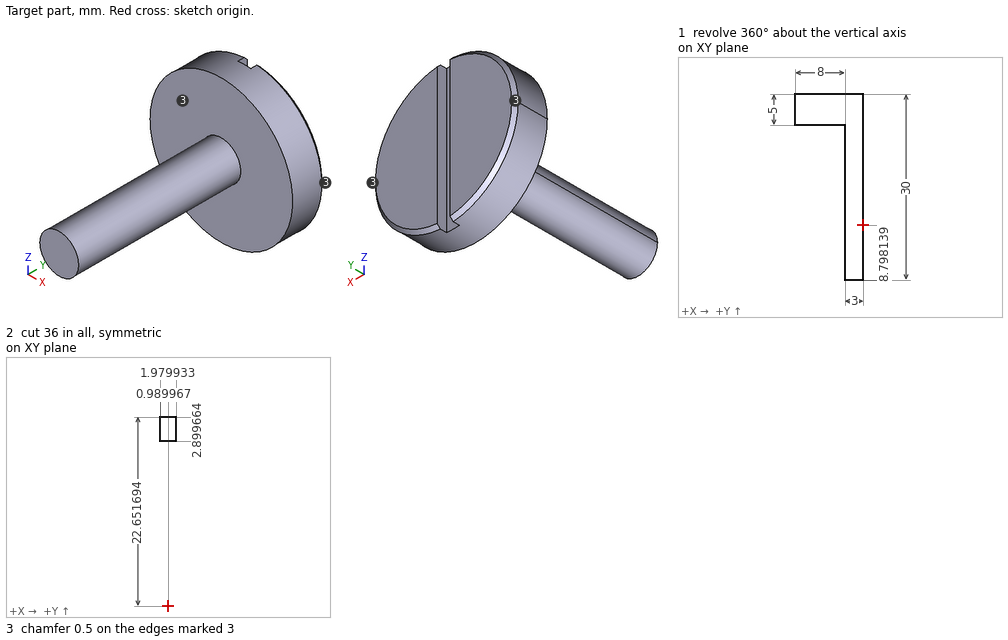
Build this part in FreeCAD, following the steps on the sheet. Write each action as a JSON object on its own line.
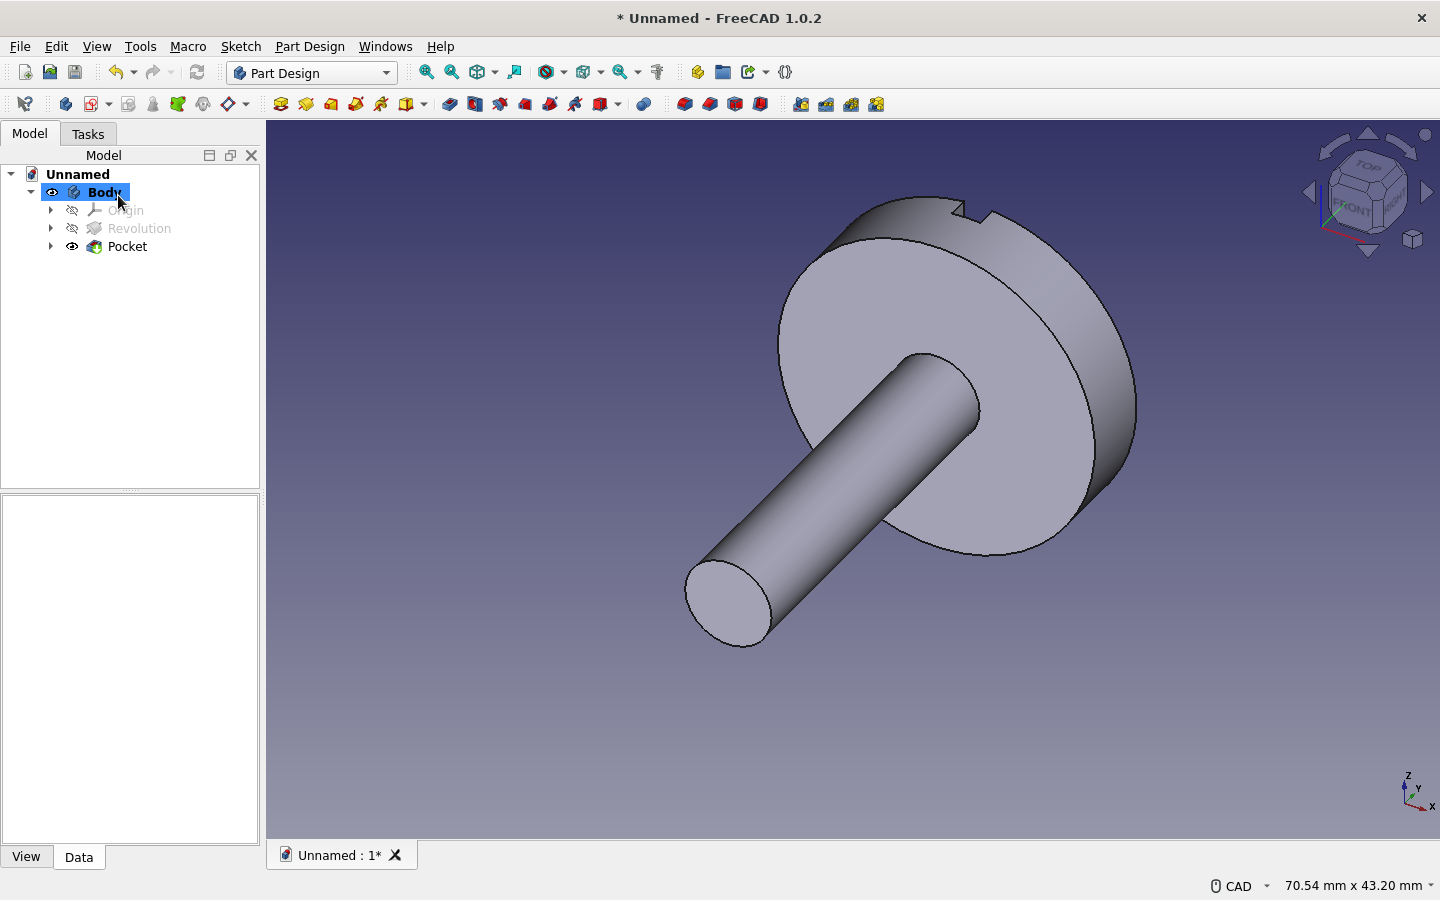
{"action": "key", "text": "0"}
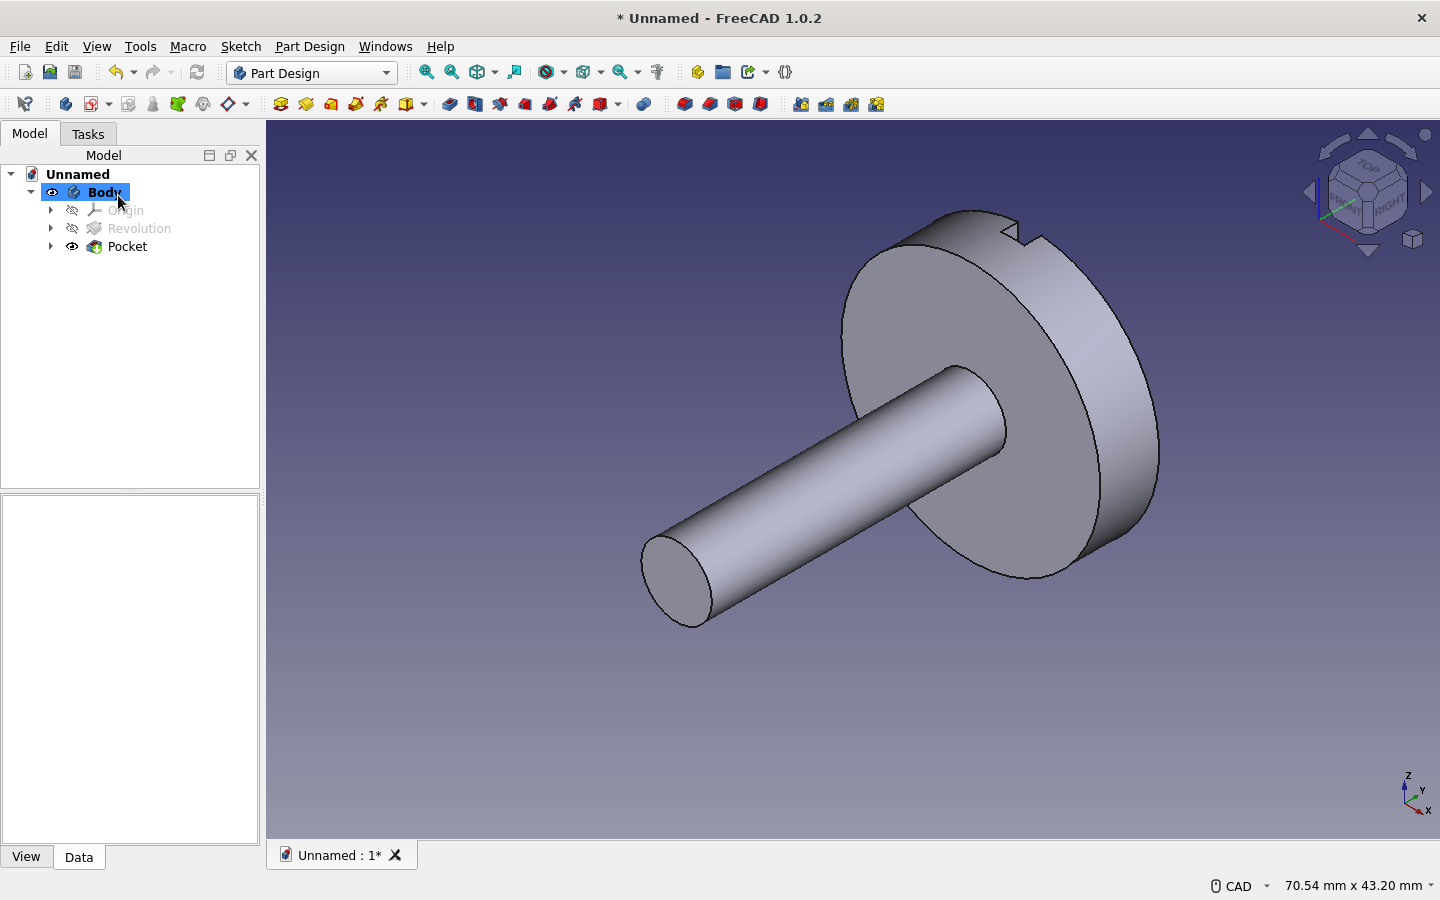
{"action": "key", "text": "2"}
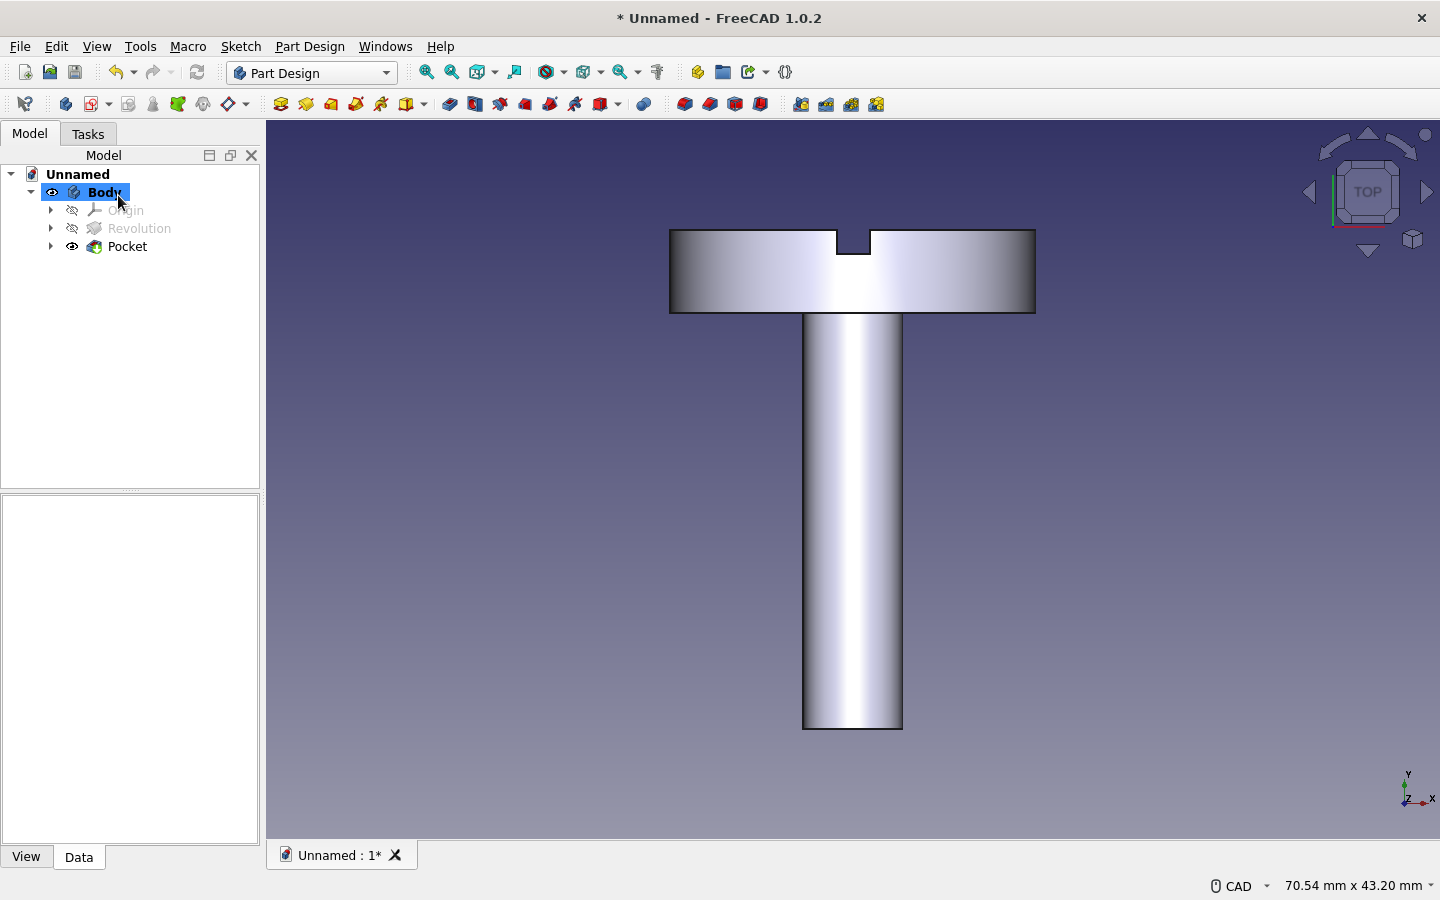
{"action": "left_click", "coordinate": [886, 229]}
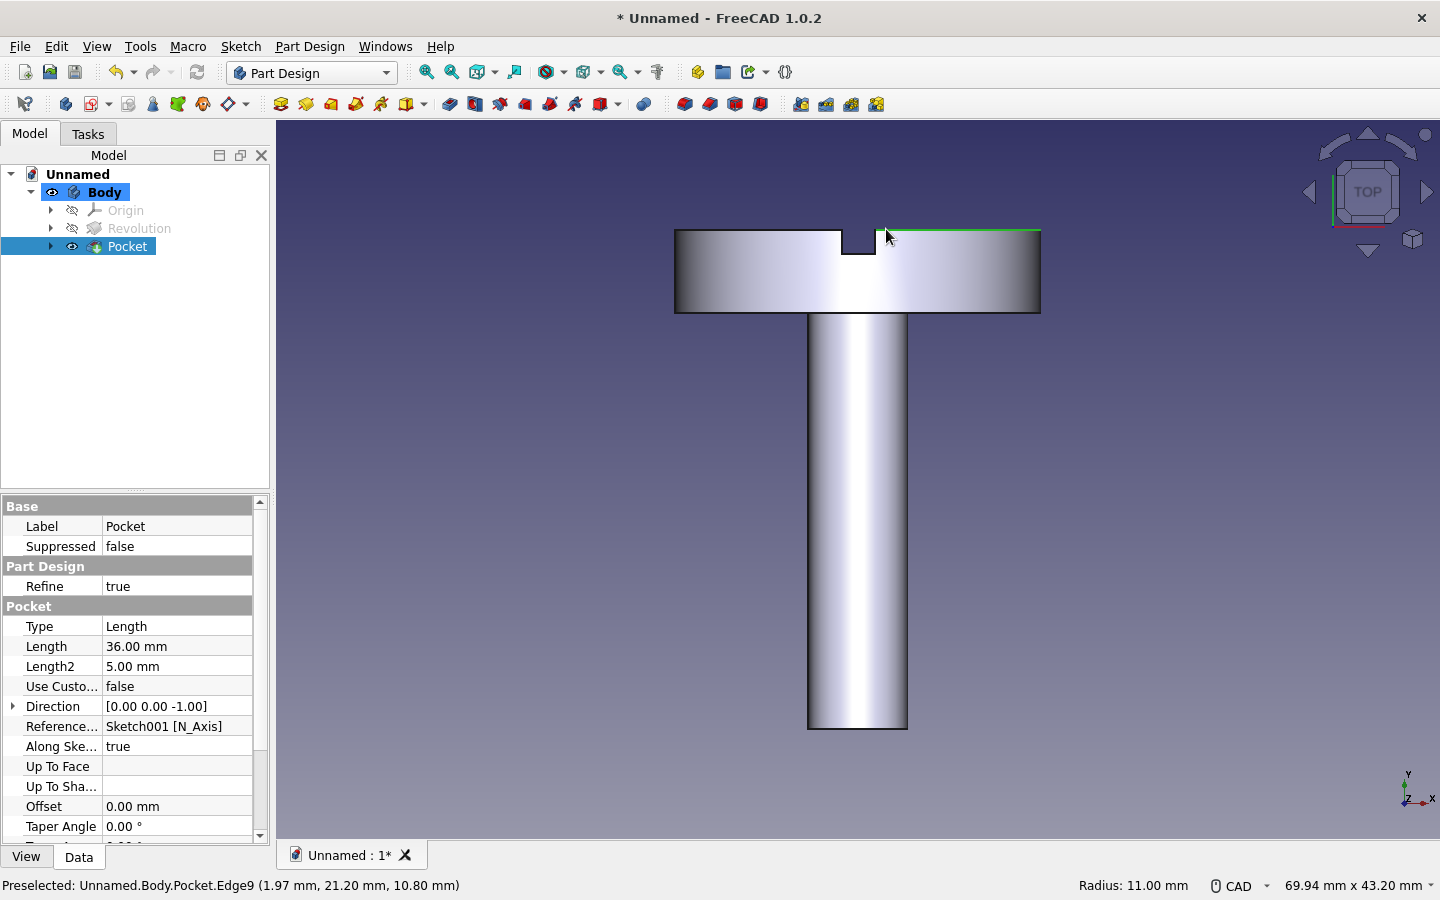
{"action": "key", "text": "1"}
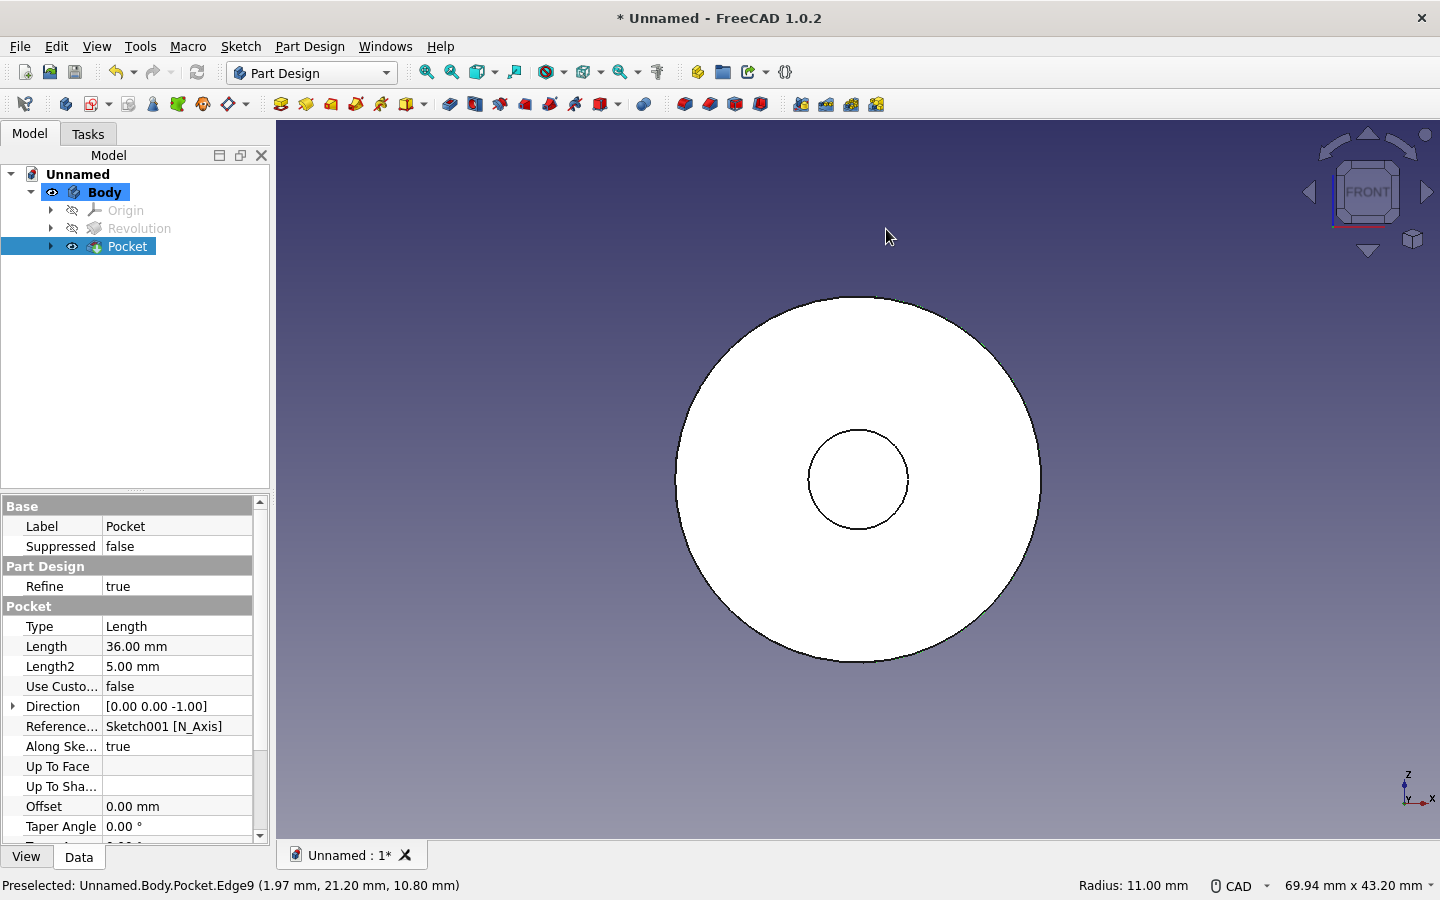
{"action": "key", "text": "3"}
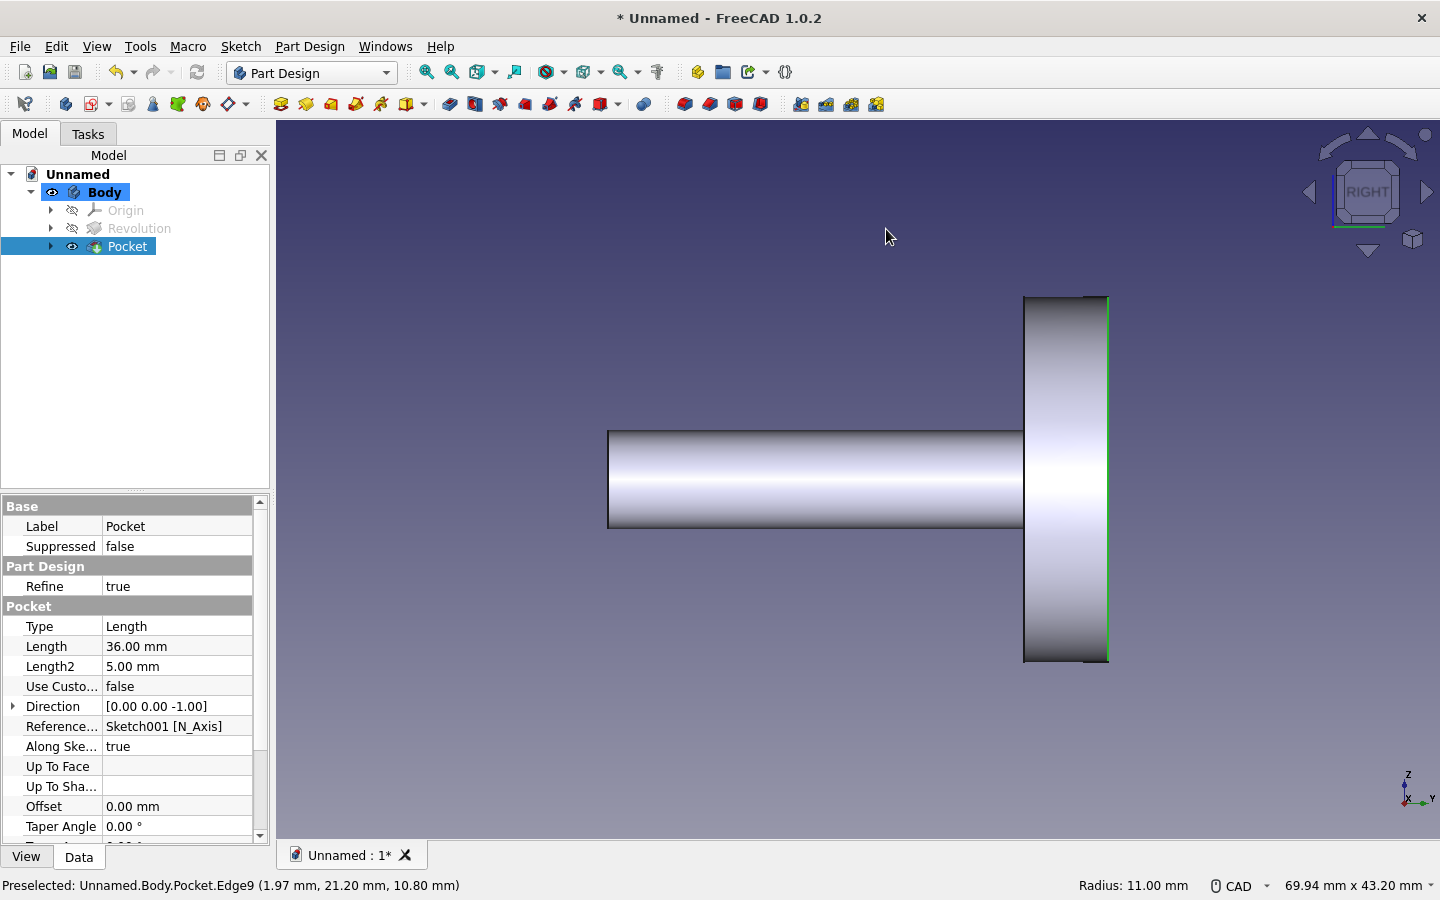
{"action": "key", "text": "5"}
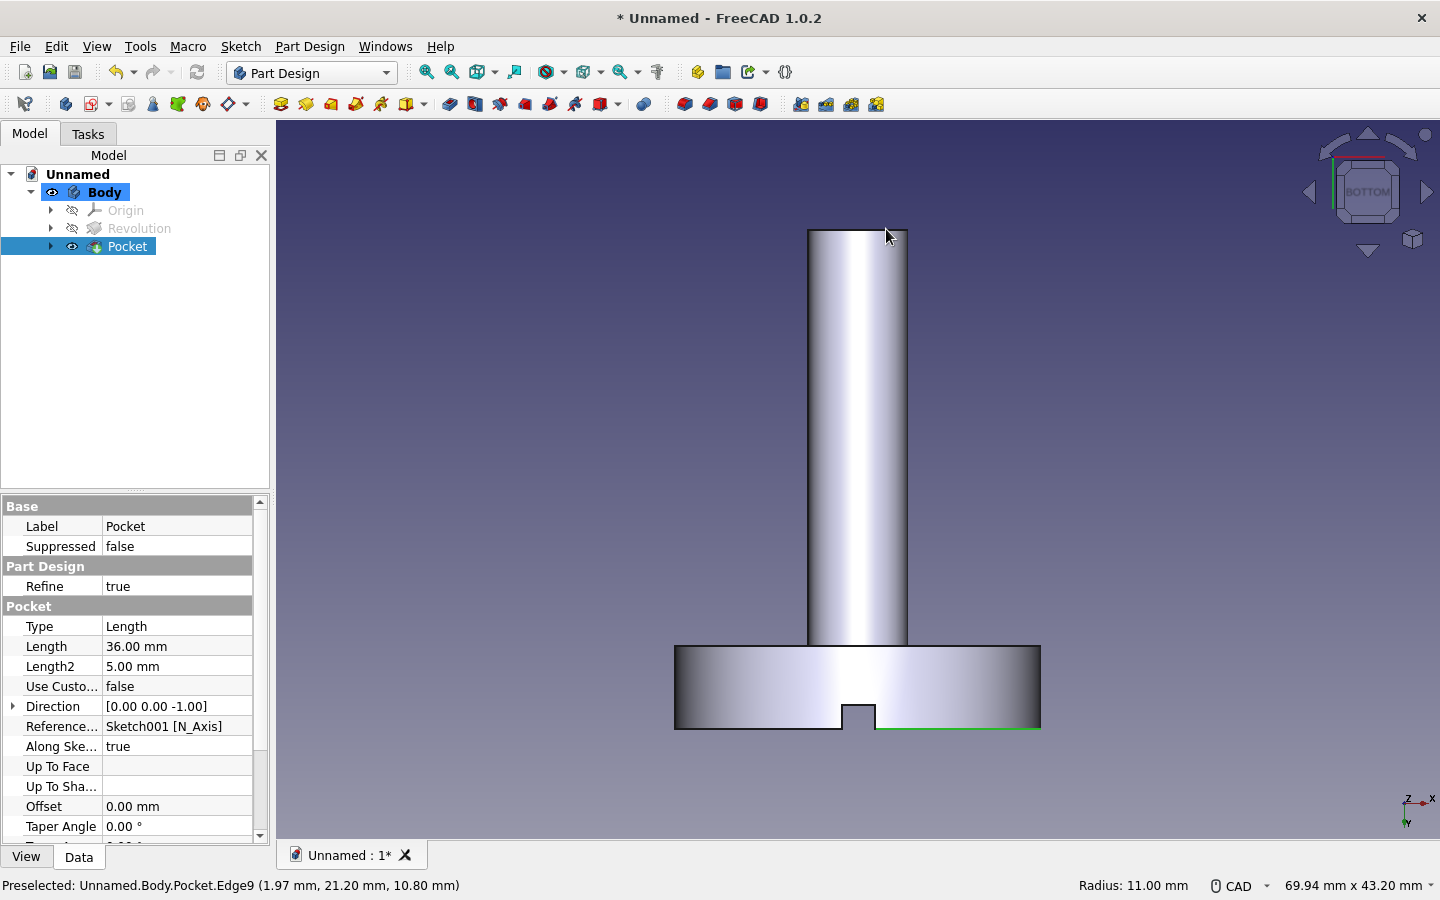
{"action": "key", "text": "4"}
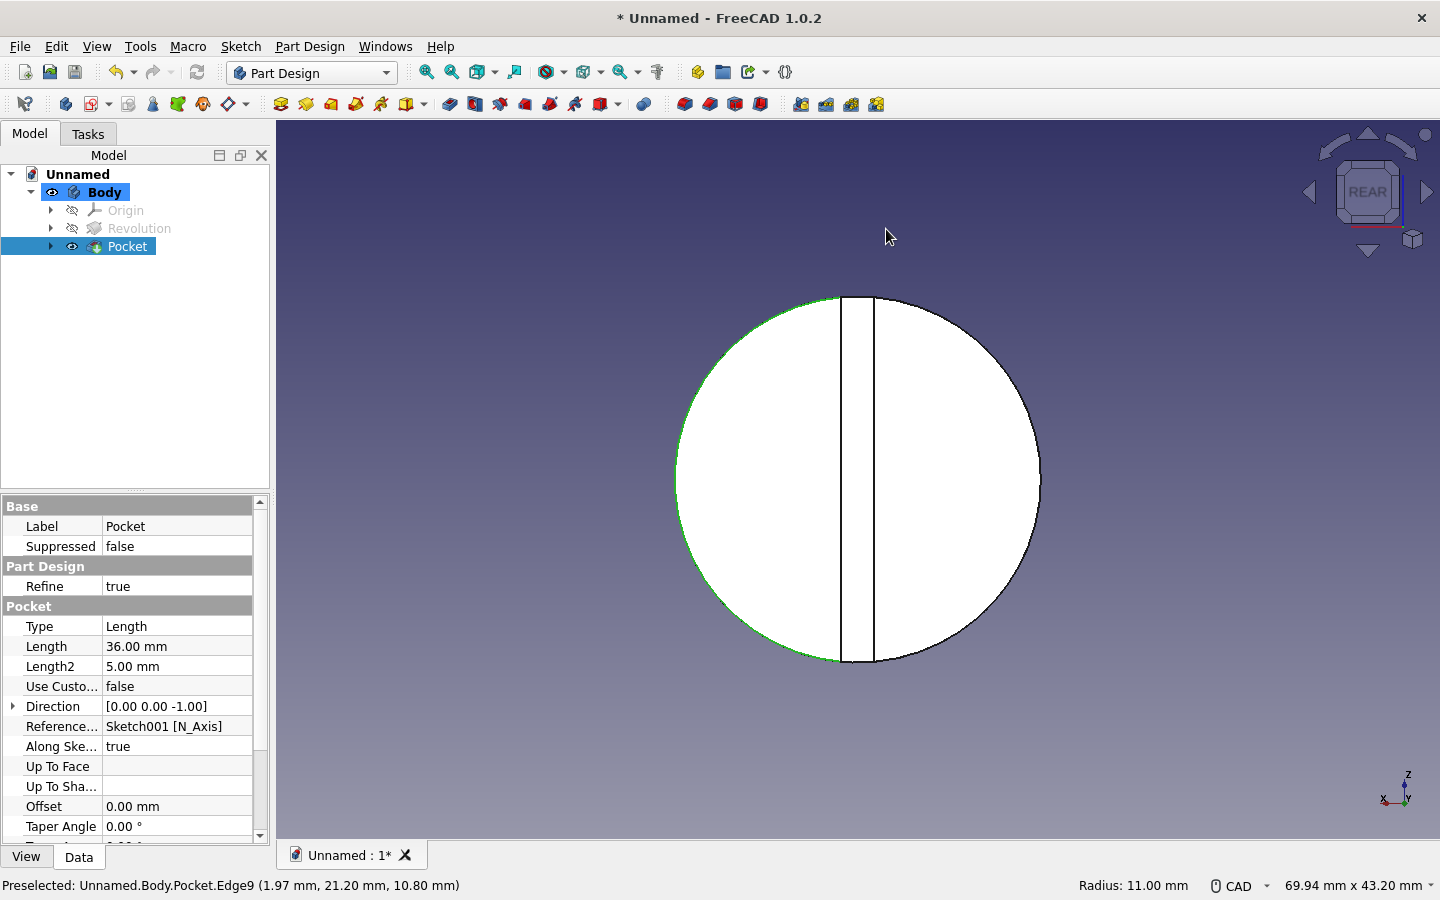
{"action": "left_click", "coordinate": [993, 355], "text": "ctrl"}